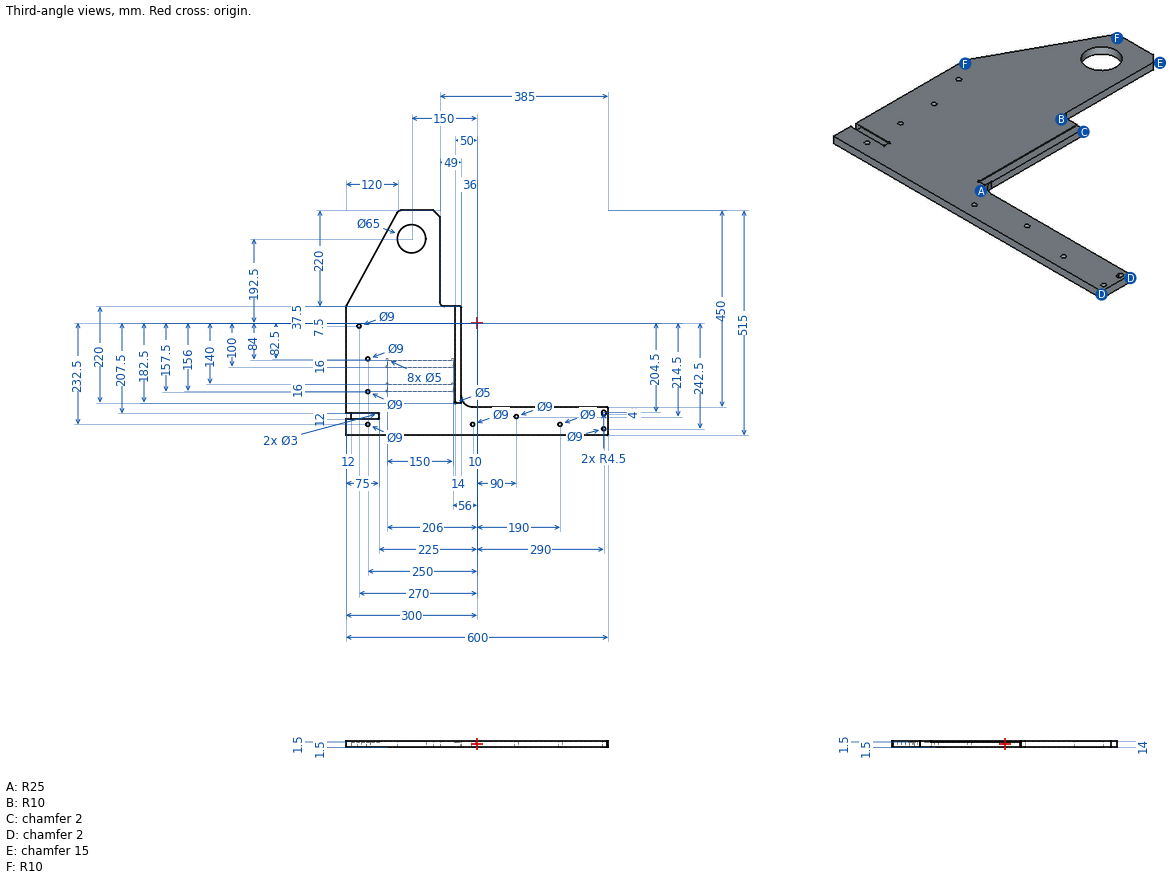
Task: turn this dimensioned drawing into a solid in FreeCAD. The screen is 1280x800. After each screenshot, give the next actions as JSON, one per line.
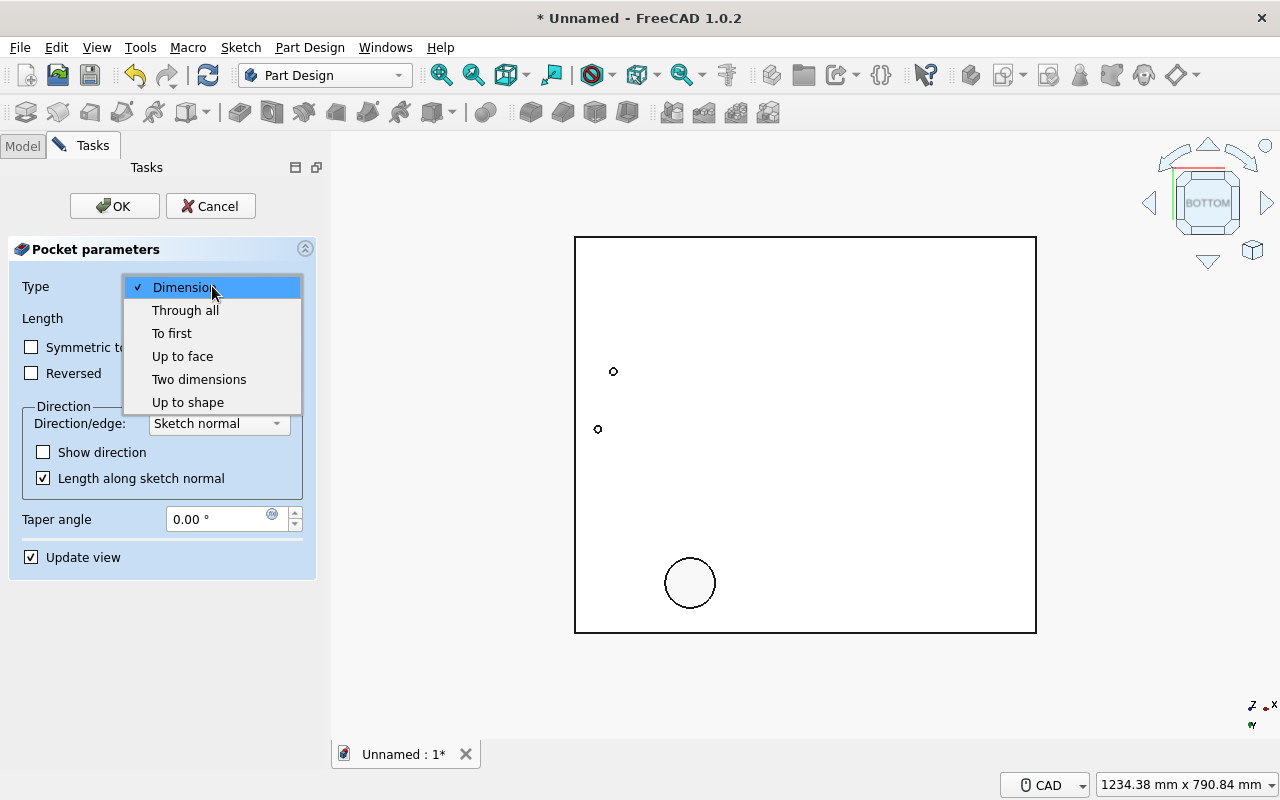
{"action": "left_click", "coordinate": [212, 334]}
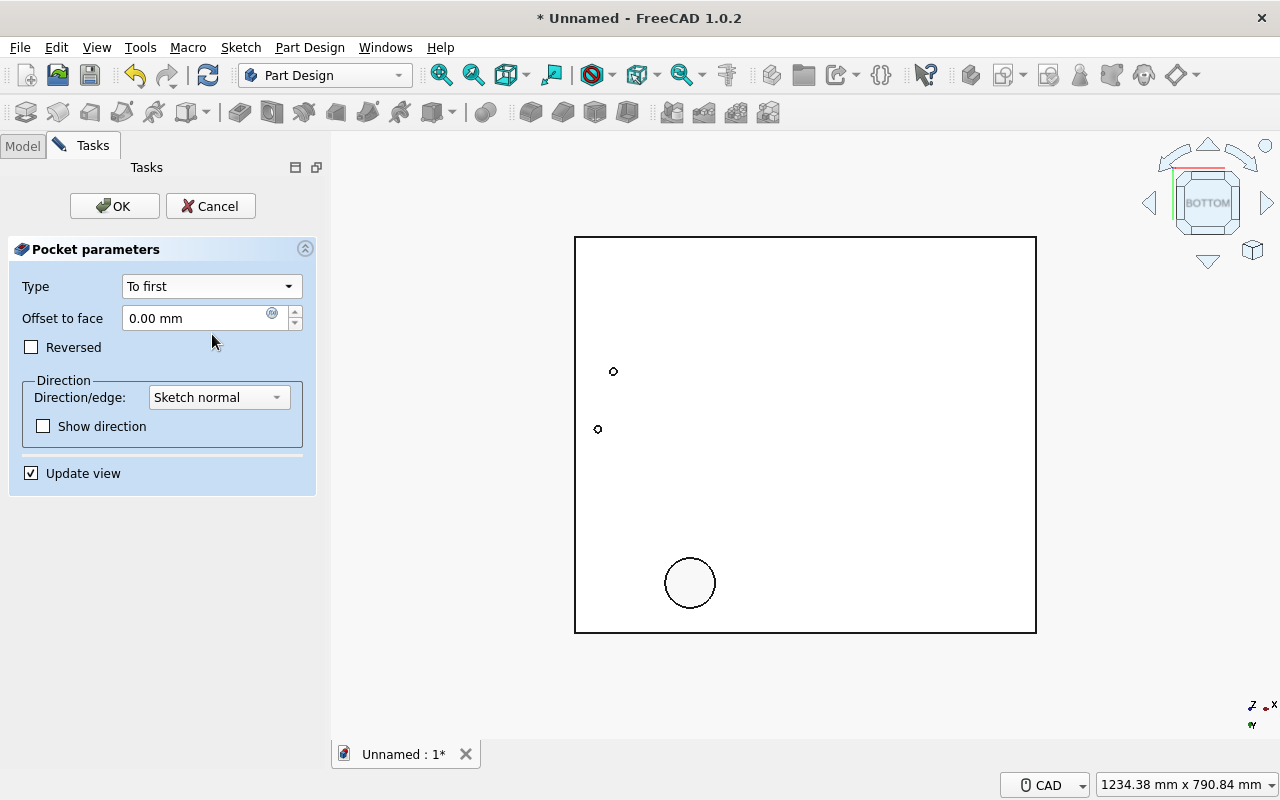
{"action": "left_click", "coordinate": [115, 206]}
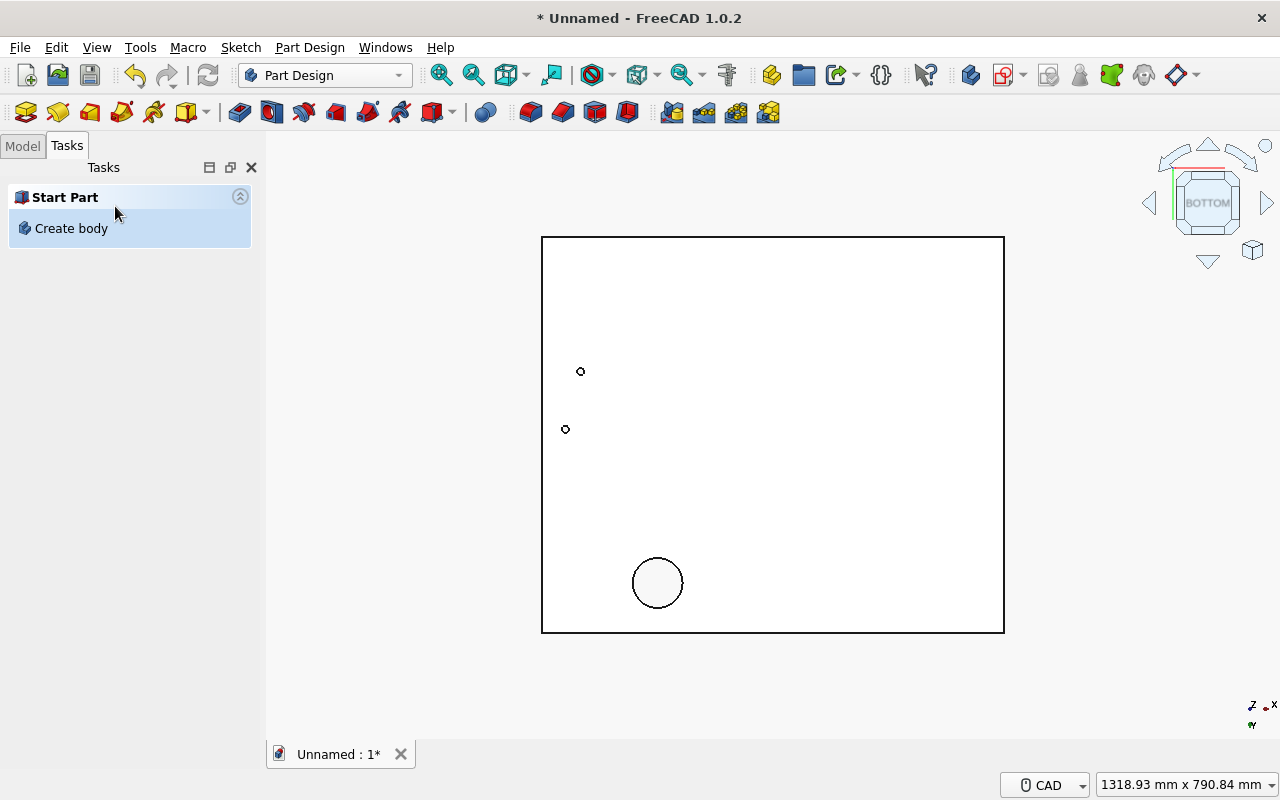
{"action": "left_click", "coordinate": [839, 434]}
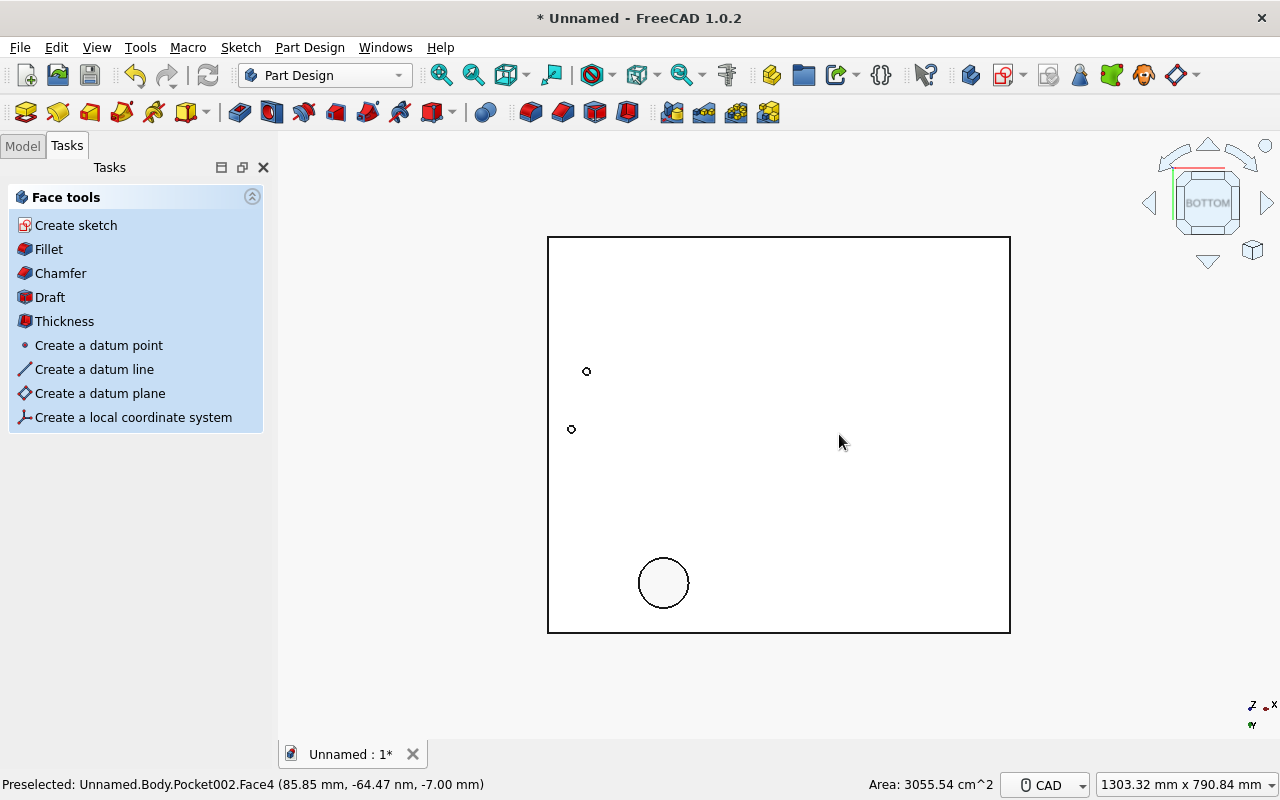
{"action": "left_click", "coordinate": [1004, 76]}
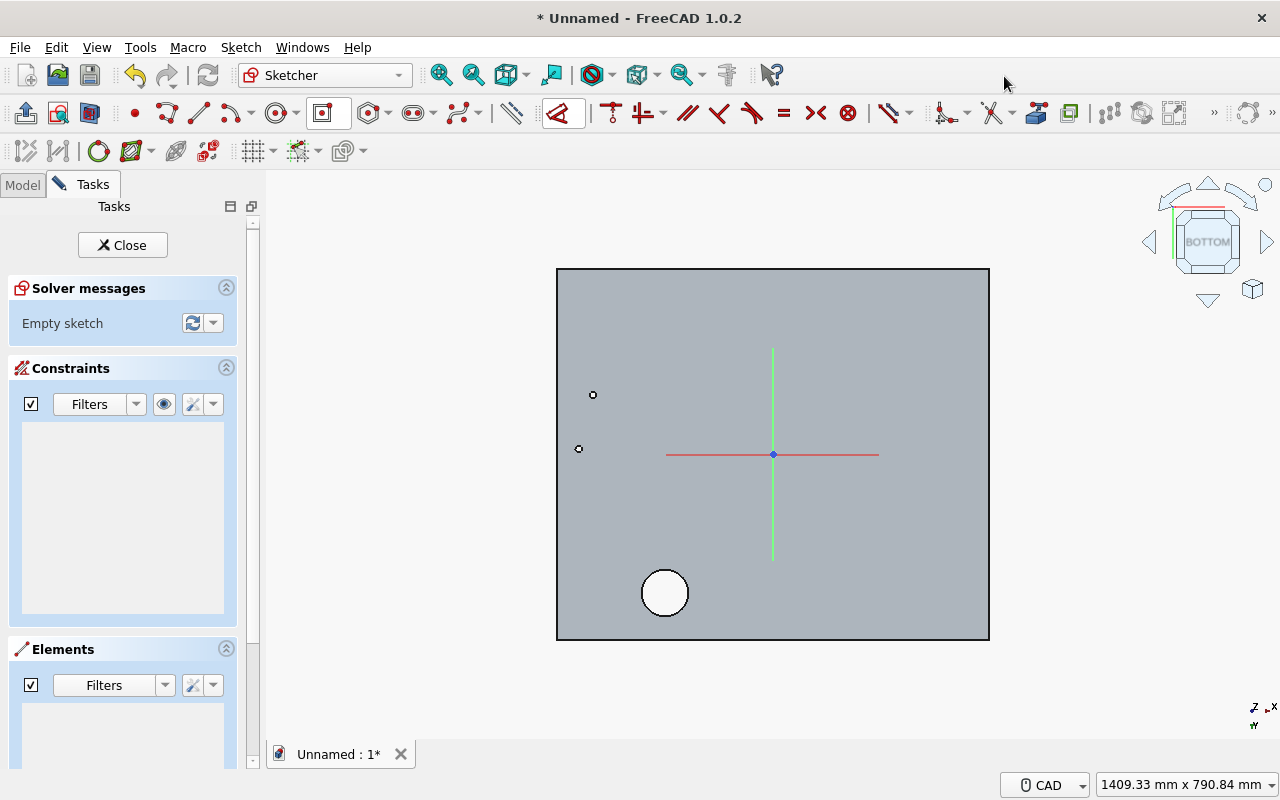
{"action": "scroll", "coordinate": [587, 335], "scroll_direction": "up", "scroll_amount": 15}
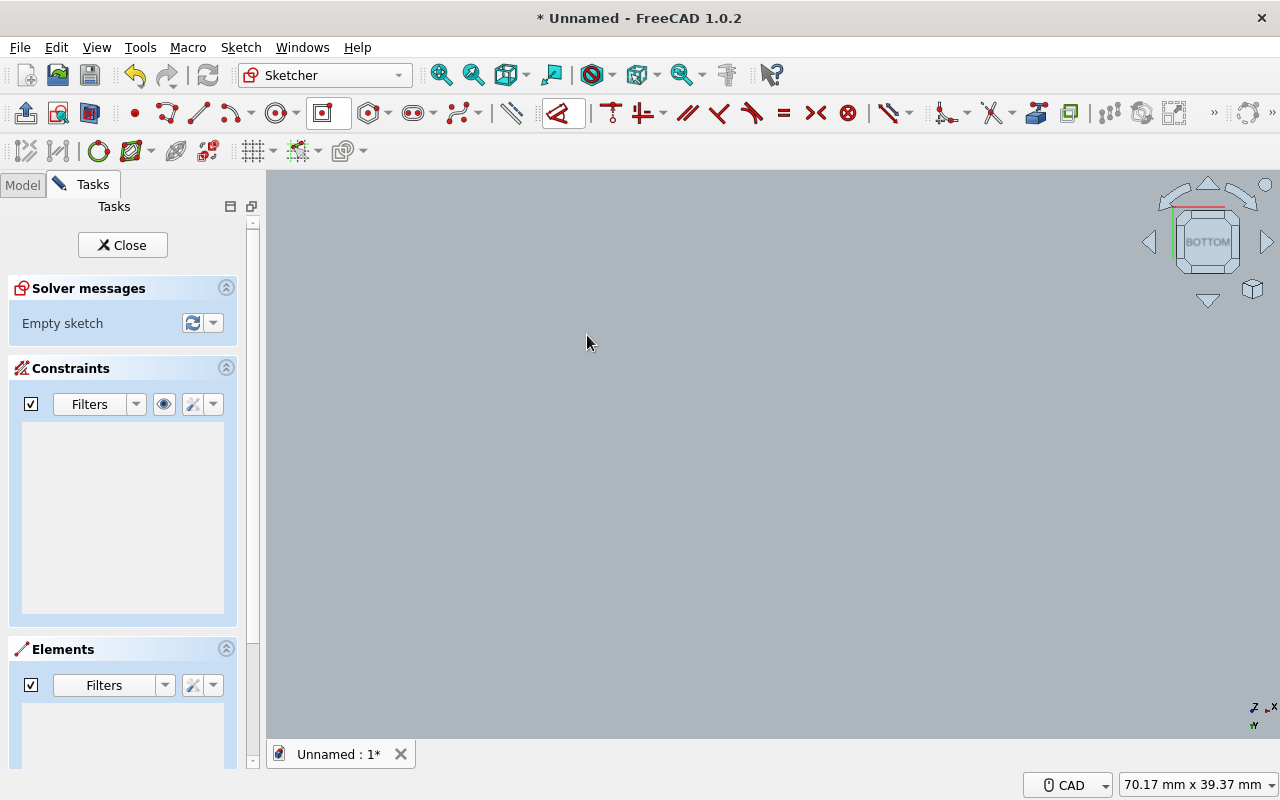
{"action": "scroll", "coordinate": [704, 453], "scroll_direction": "up", "scroll_amount": 5}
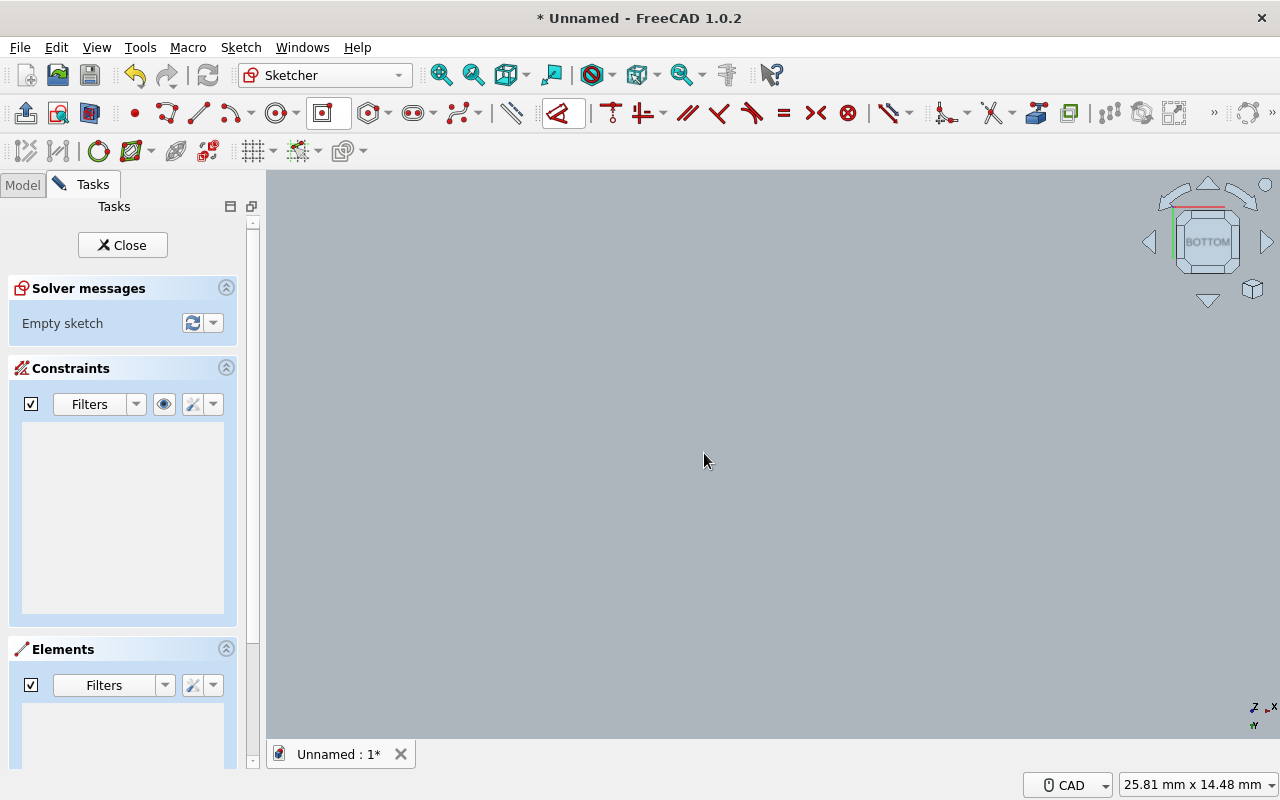
{"action": "left_click", "coordinate": [276, 114]}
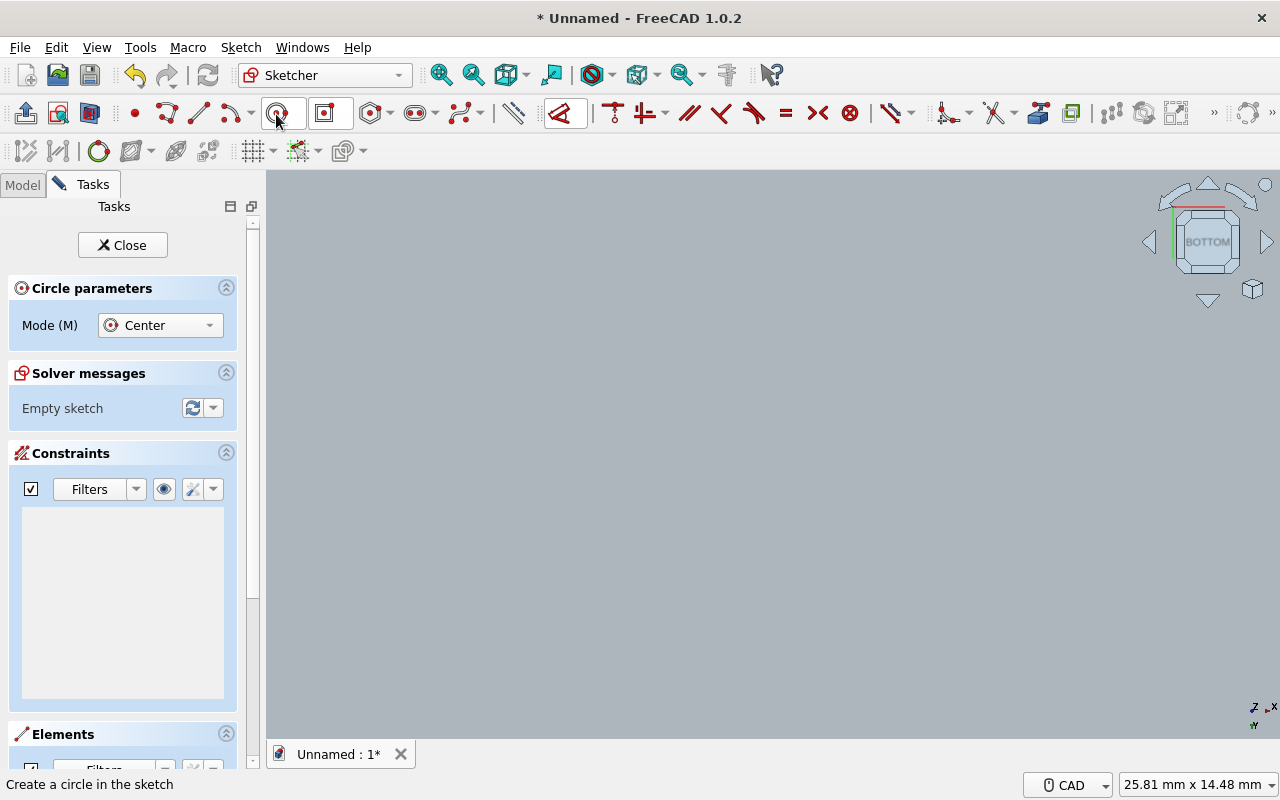
{"action": "left_click", "coordinate": [703, 454]}
{"action": "mouse_move", "coordinate": [828, 329]}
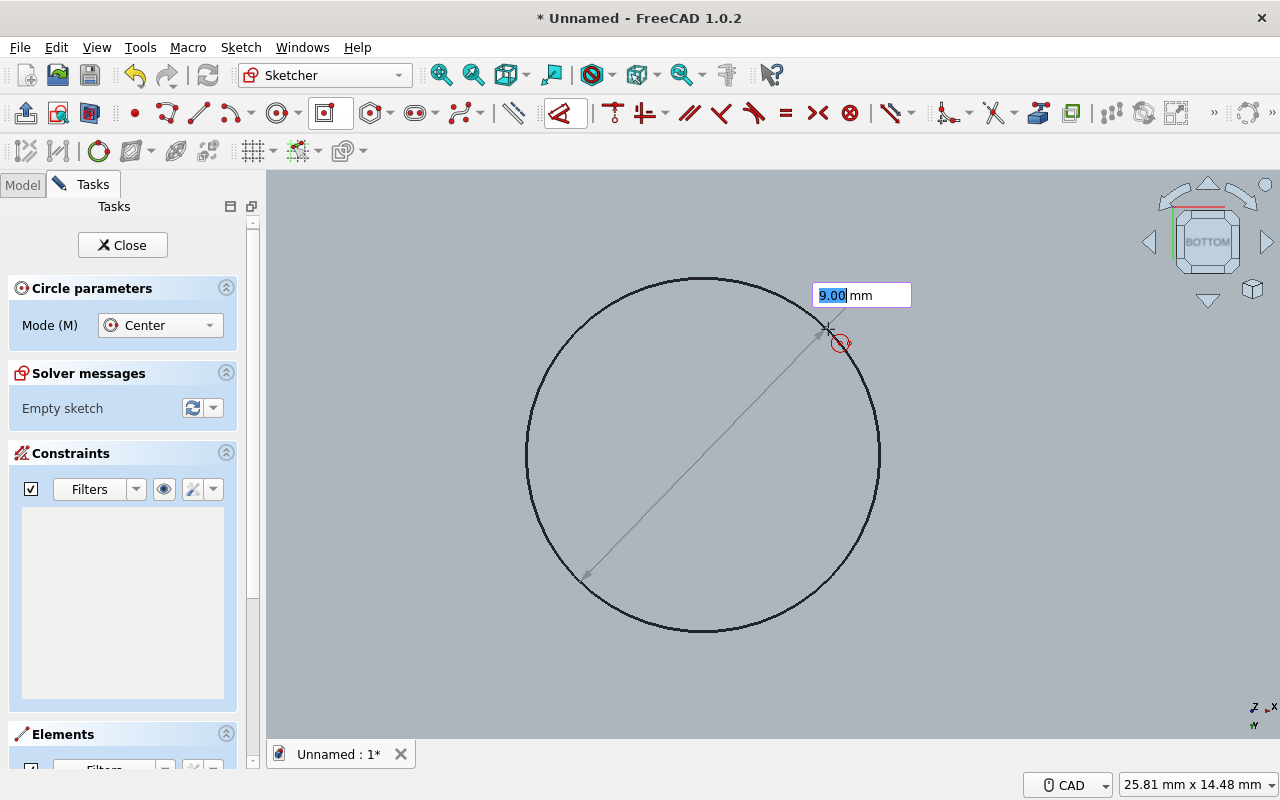
{"action": "type", "text": "9"}
{"action": "key", "text": "Return"}
{"action": "key", "text": "Escape"}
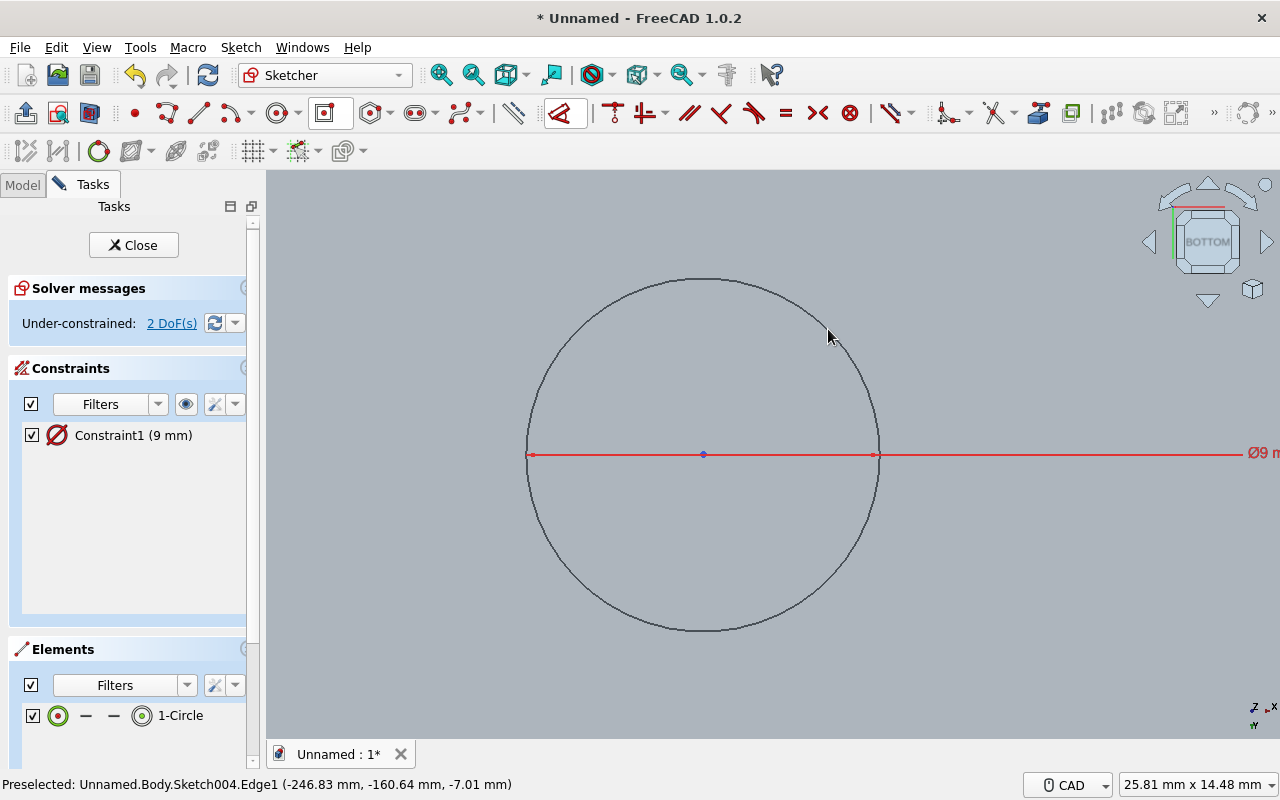
{"action": "left_click", "coordinate": [703, 455]}